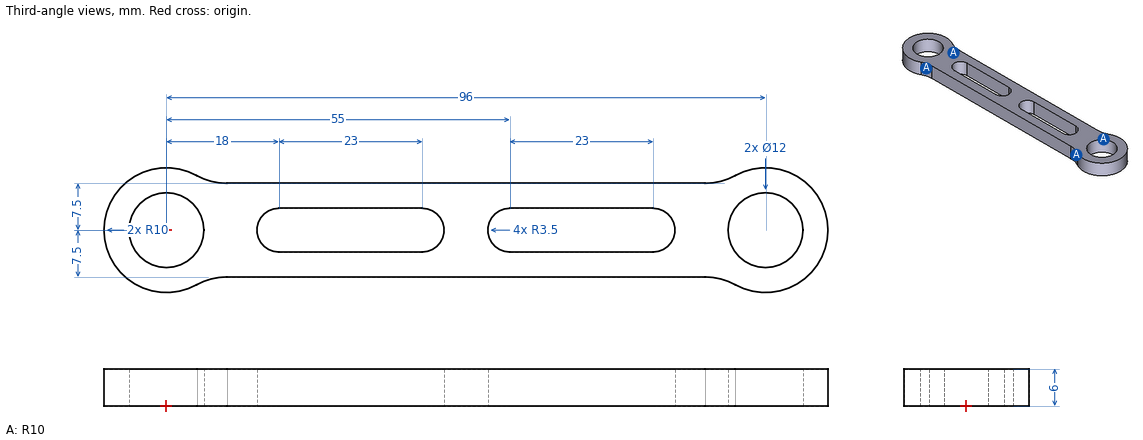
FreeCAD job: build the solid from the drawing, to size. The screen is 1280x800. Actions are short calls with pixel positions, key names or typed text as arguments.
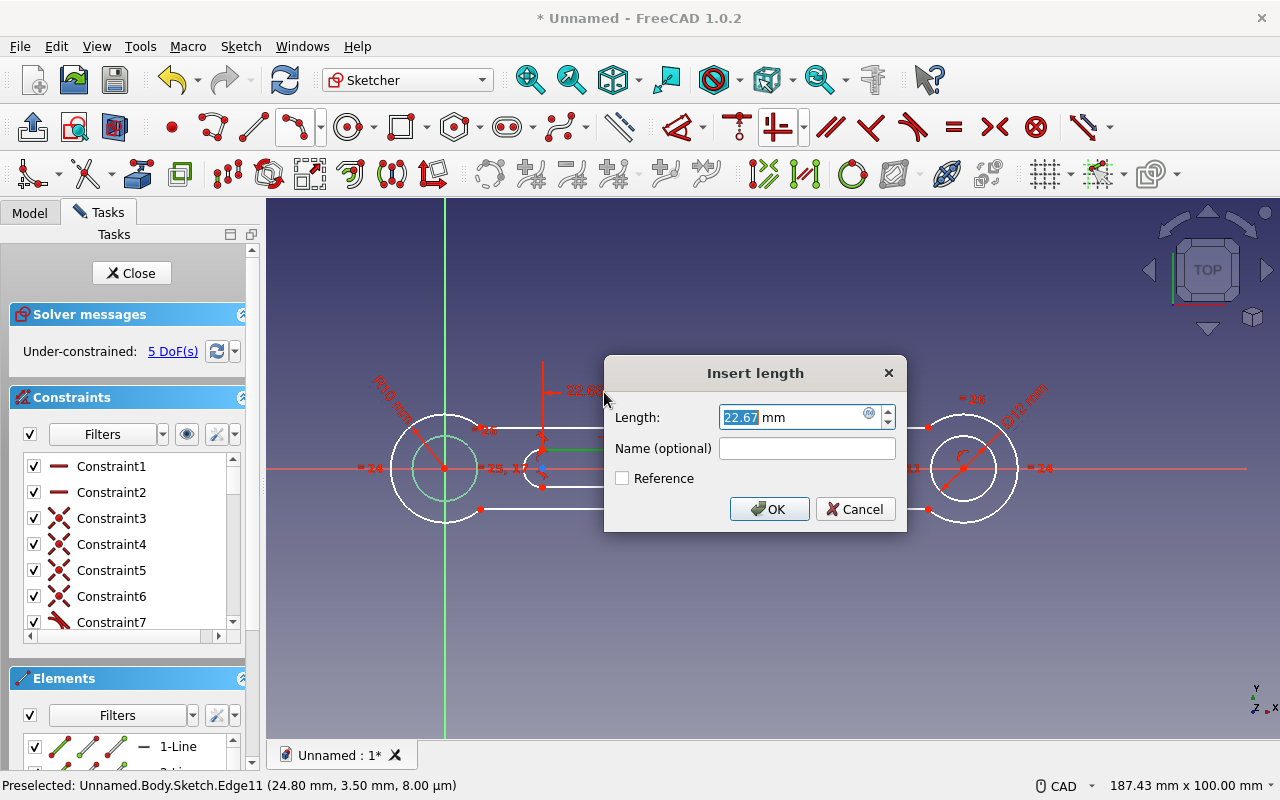
text(23)
key(Return)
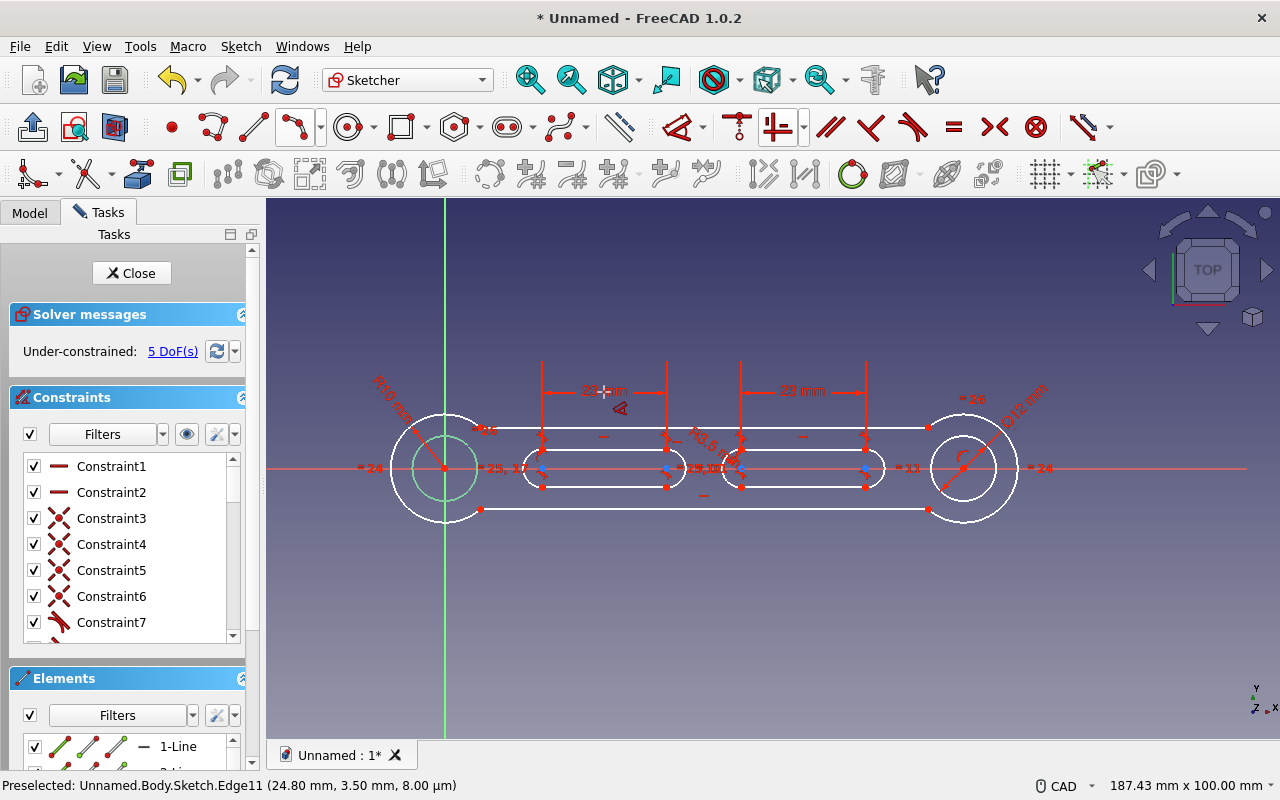
click(964, 469)
click(704, 527)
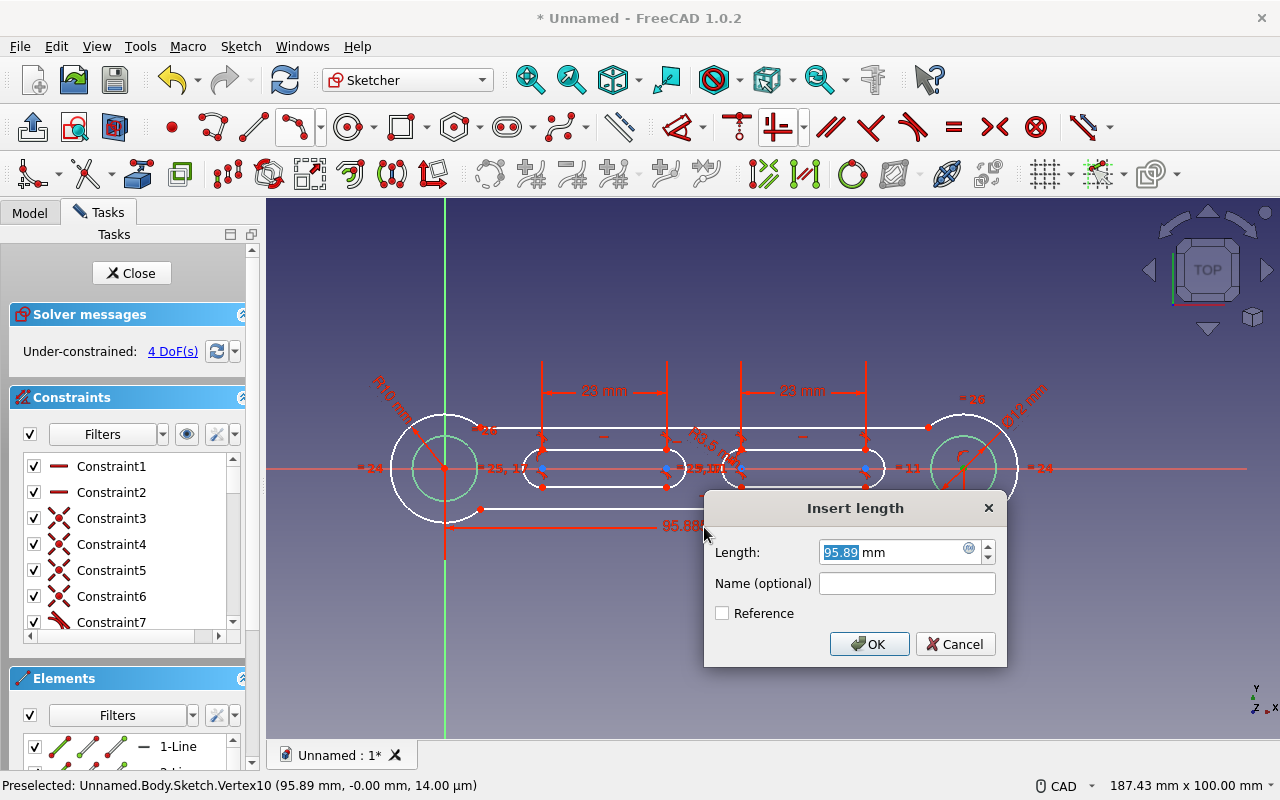
text(96)
key(Return)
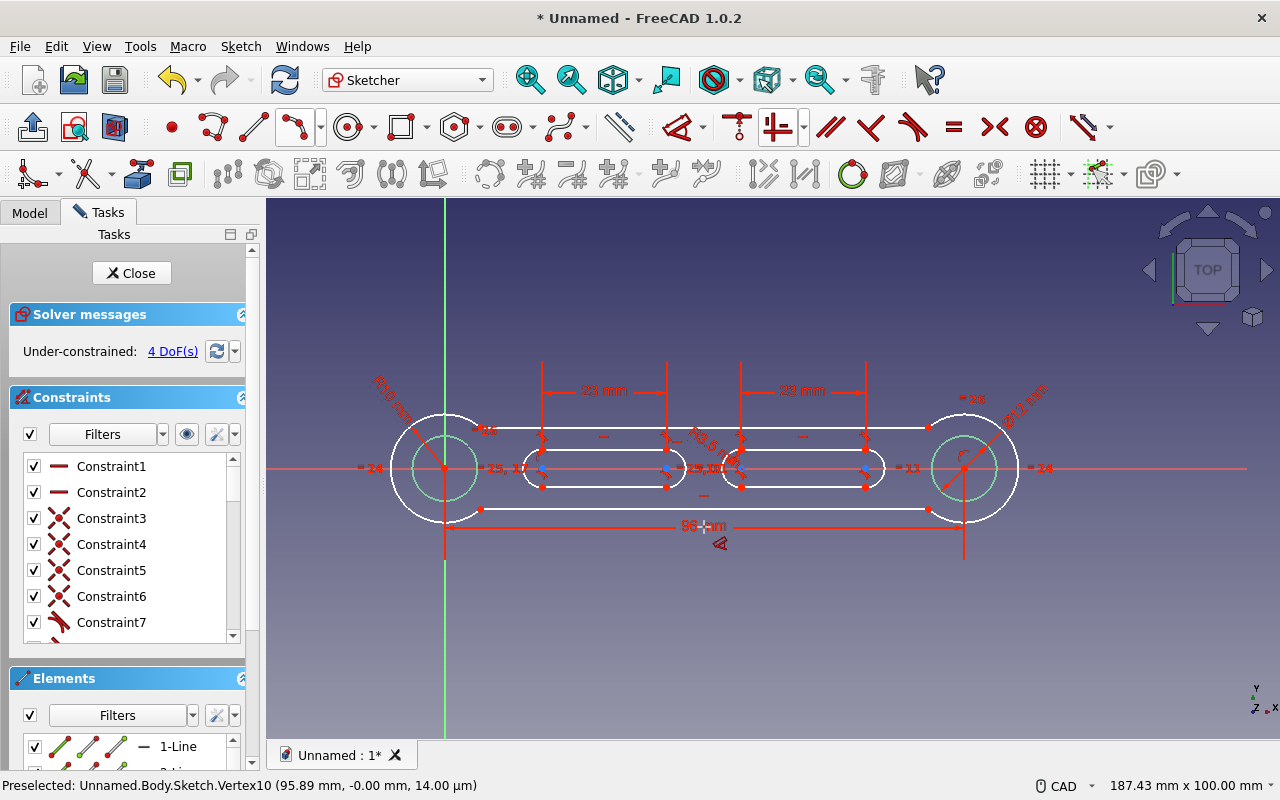
click(741, 450)
click(525, 392)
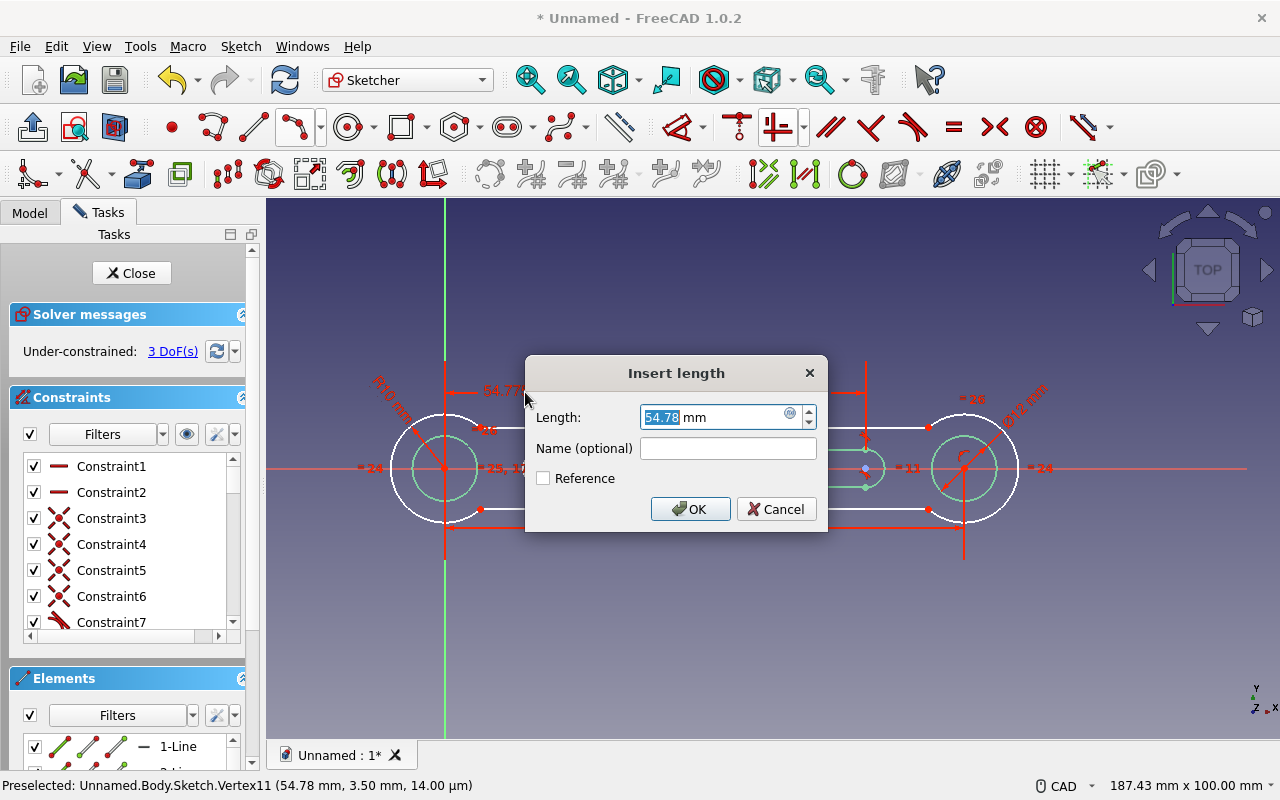
text(55)
key(Return)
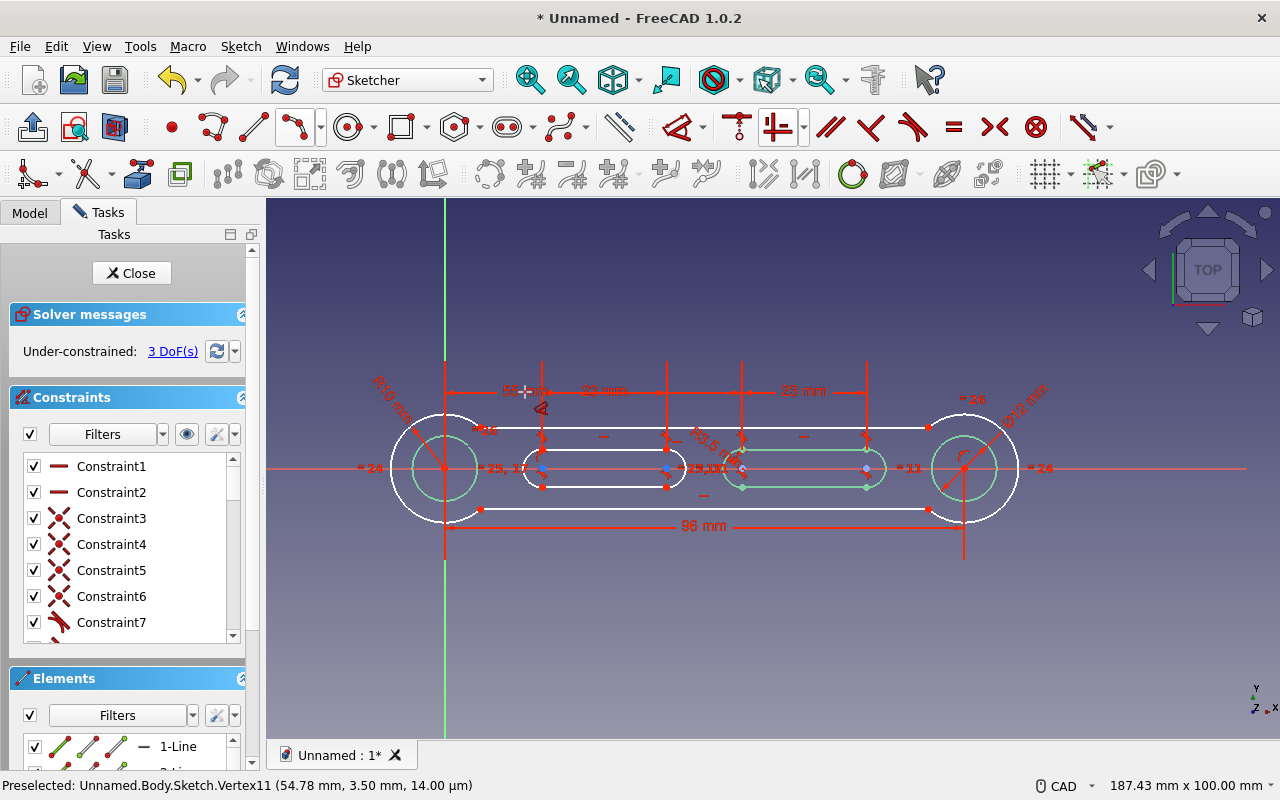
click(542, 450)
click(494, 527)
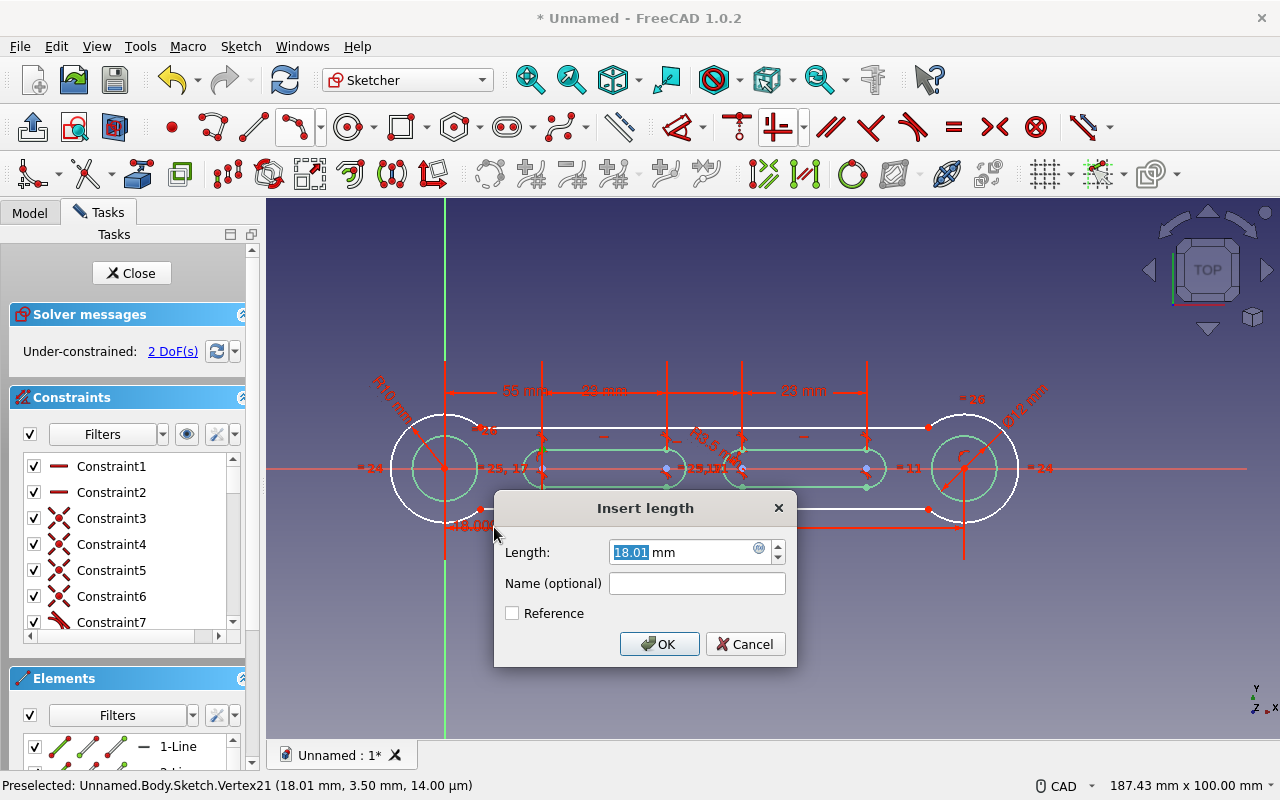
text(18)
key(Return)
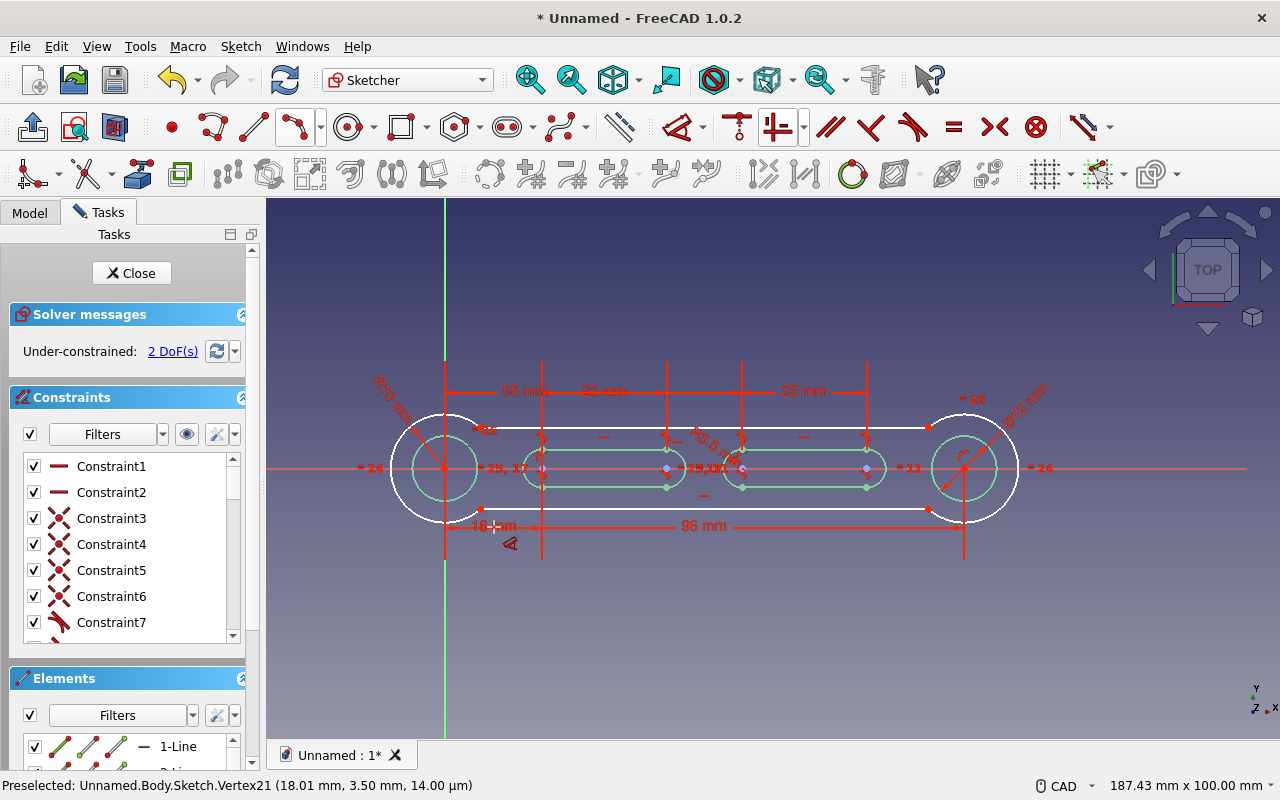
click(929, 428)
click(387, 434)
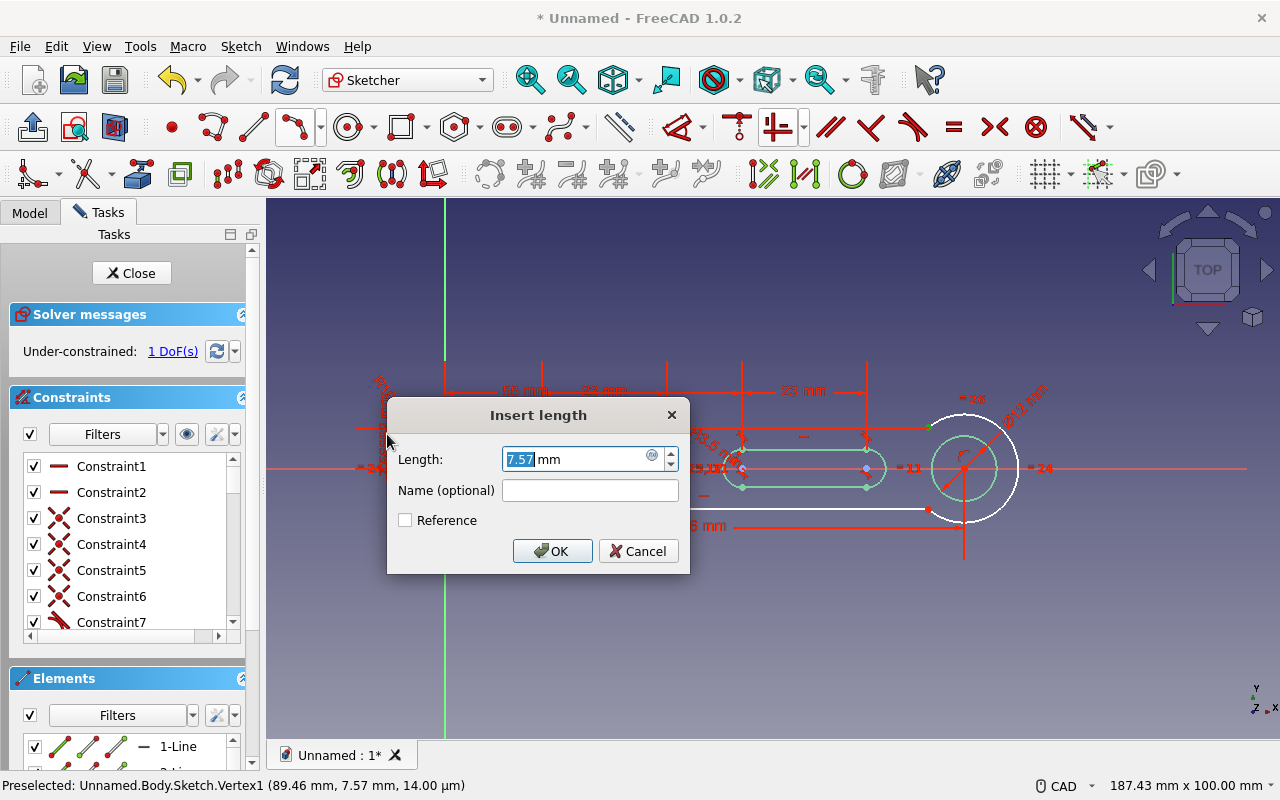
text(7.5)
key(Return)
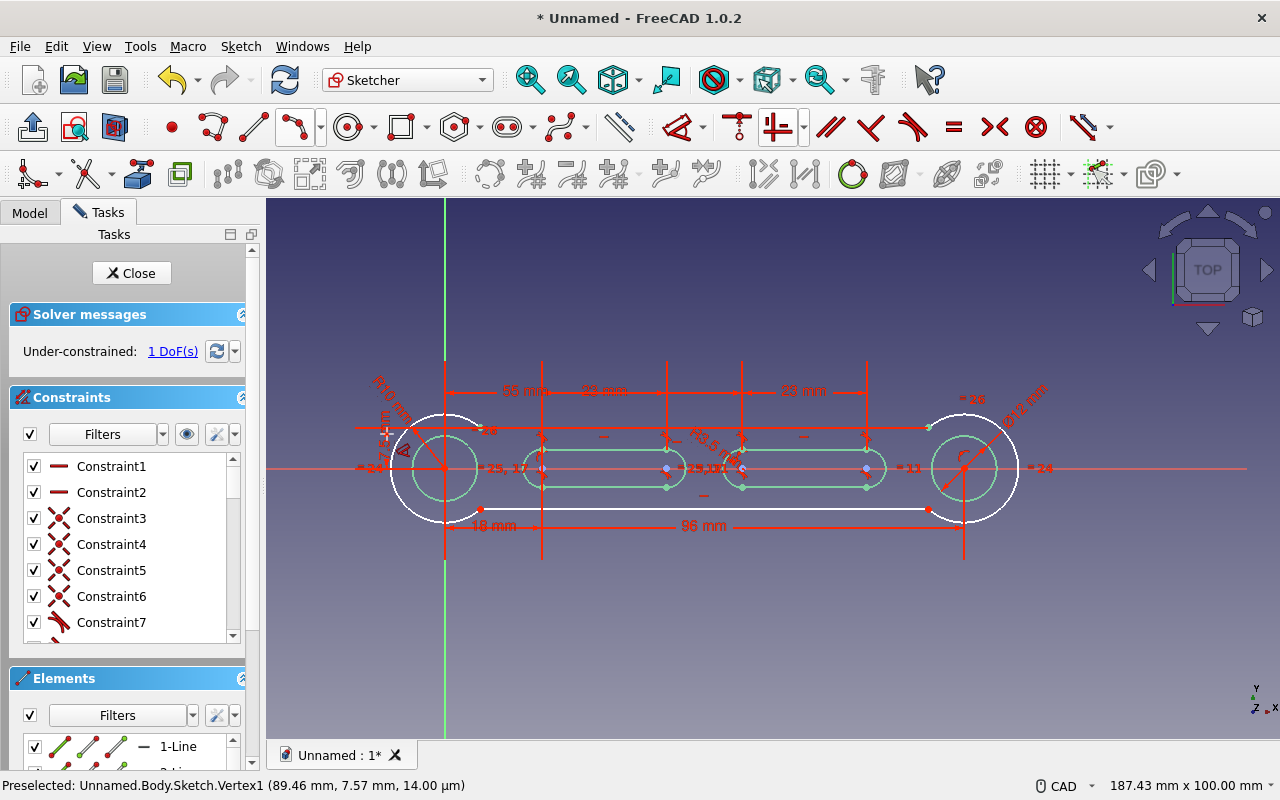
click(480, 509)
click(514, 489)